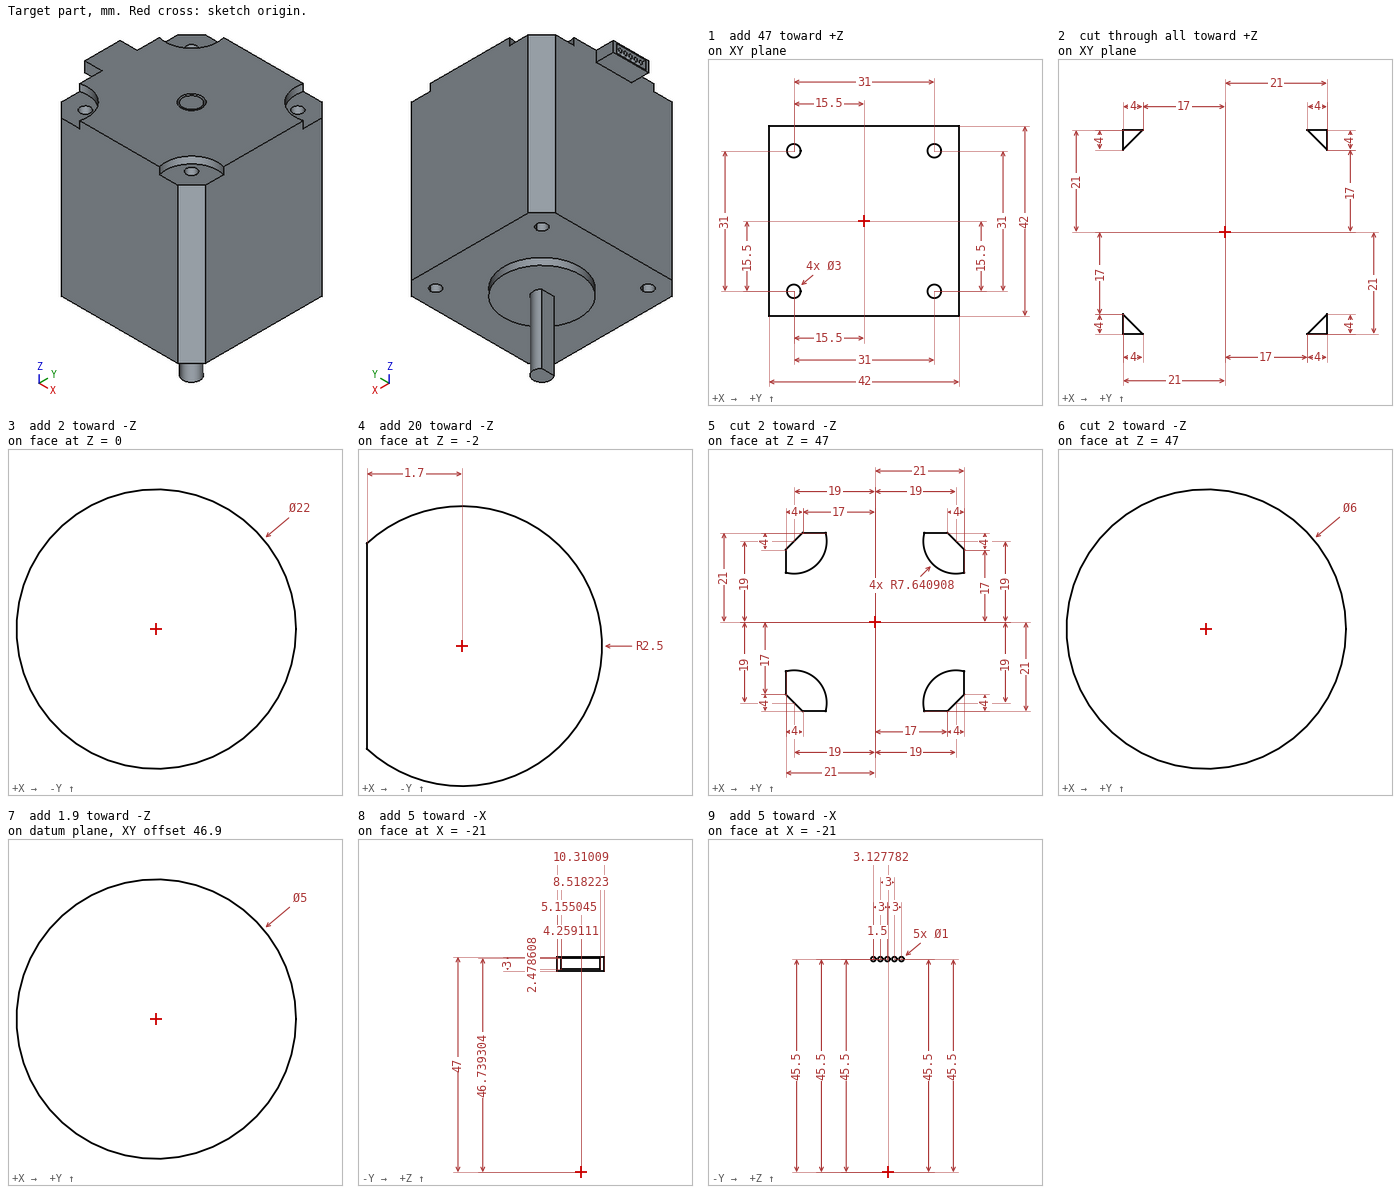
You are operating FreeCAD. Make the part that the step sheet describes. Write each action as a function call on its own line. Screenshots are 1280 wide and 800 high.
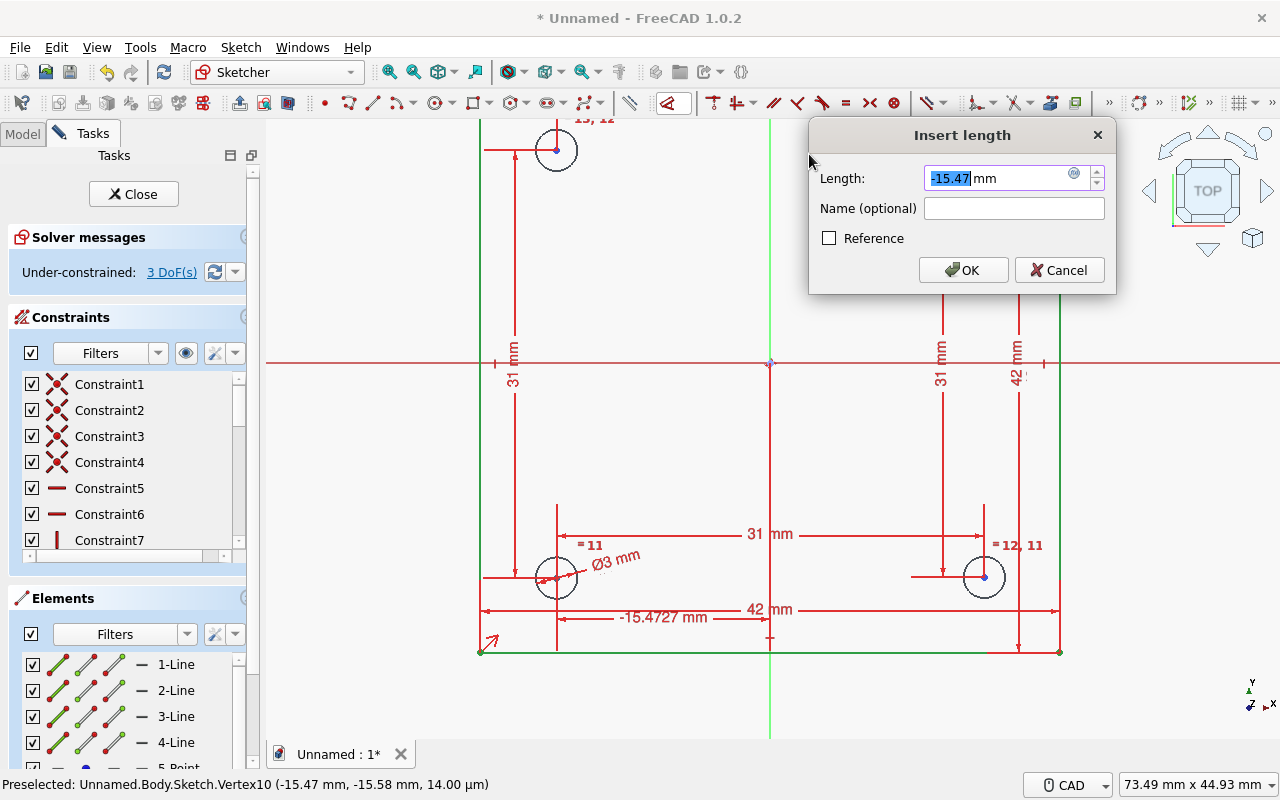
text(-15.5)
key(Return)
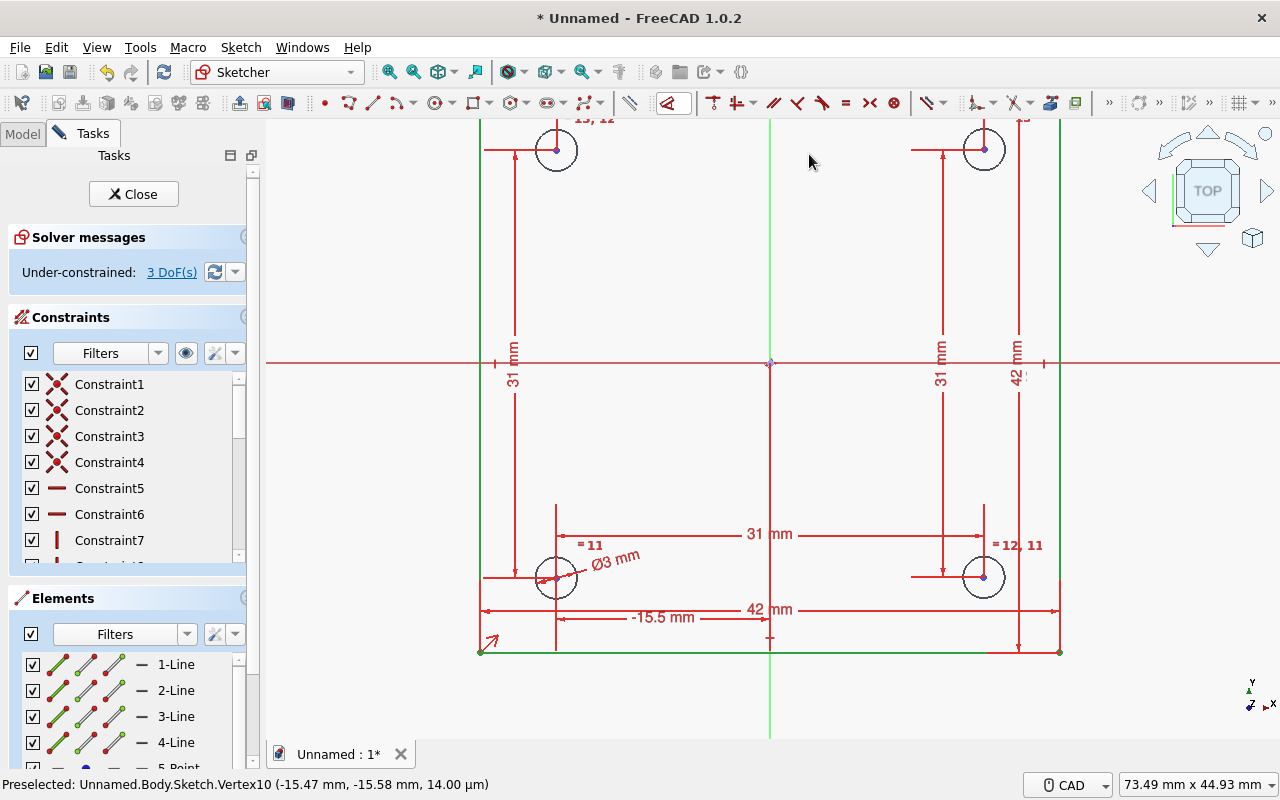
click(556, 578)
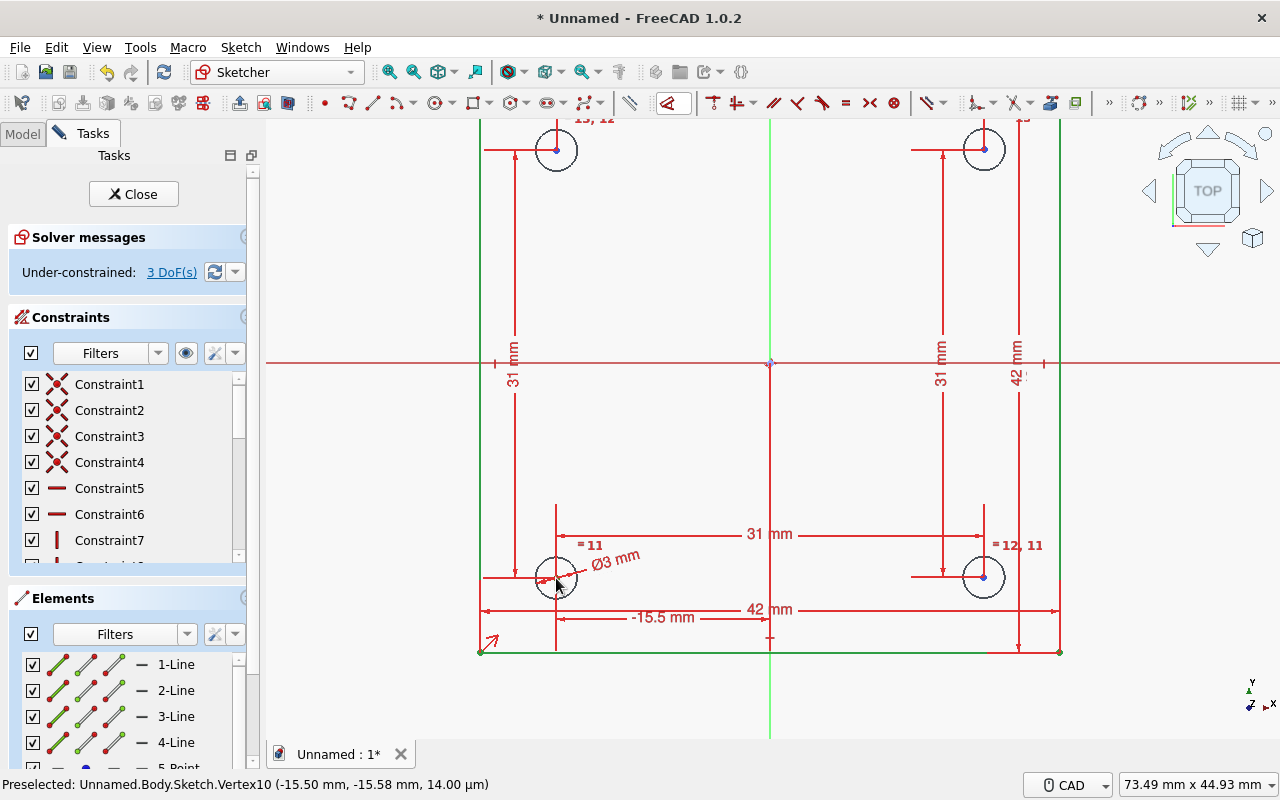
key(i)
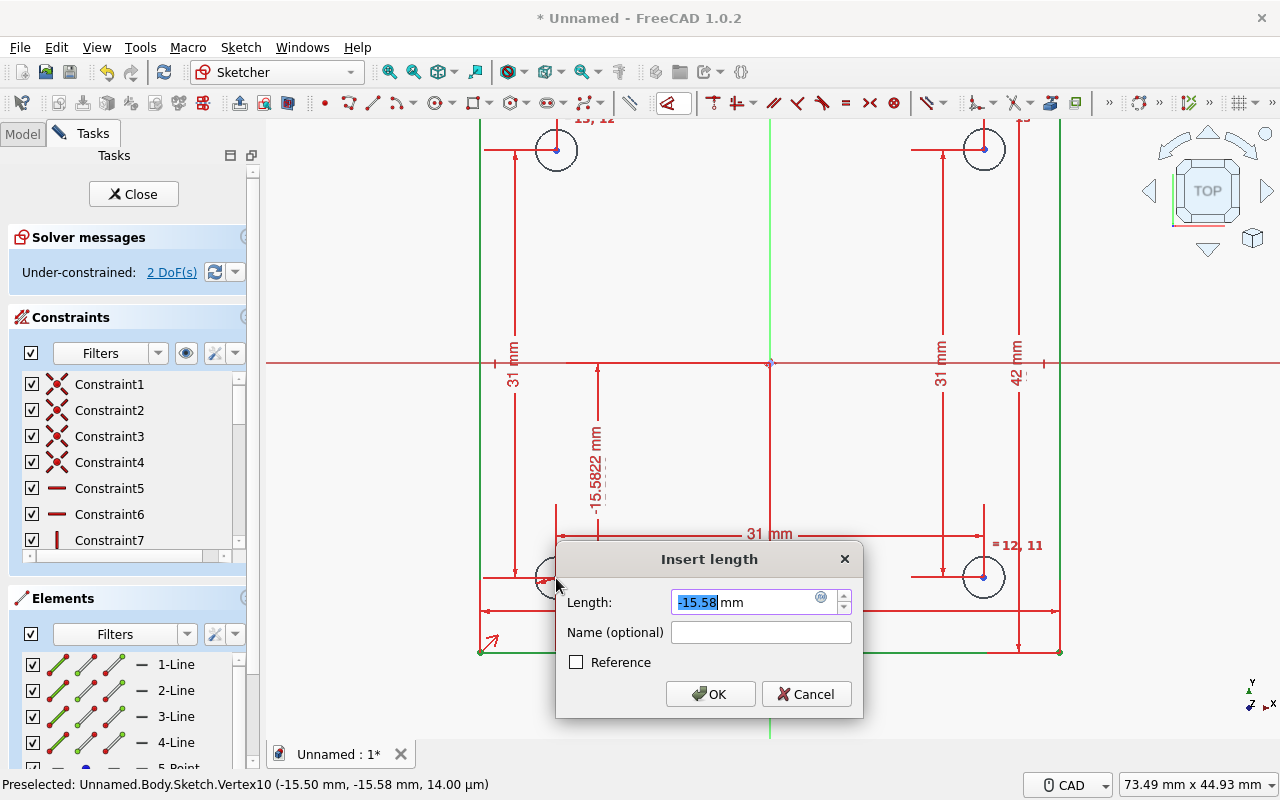
text(-15.5)
key(Return)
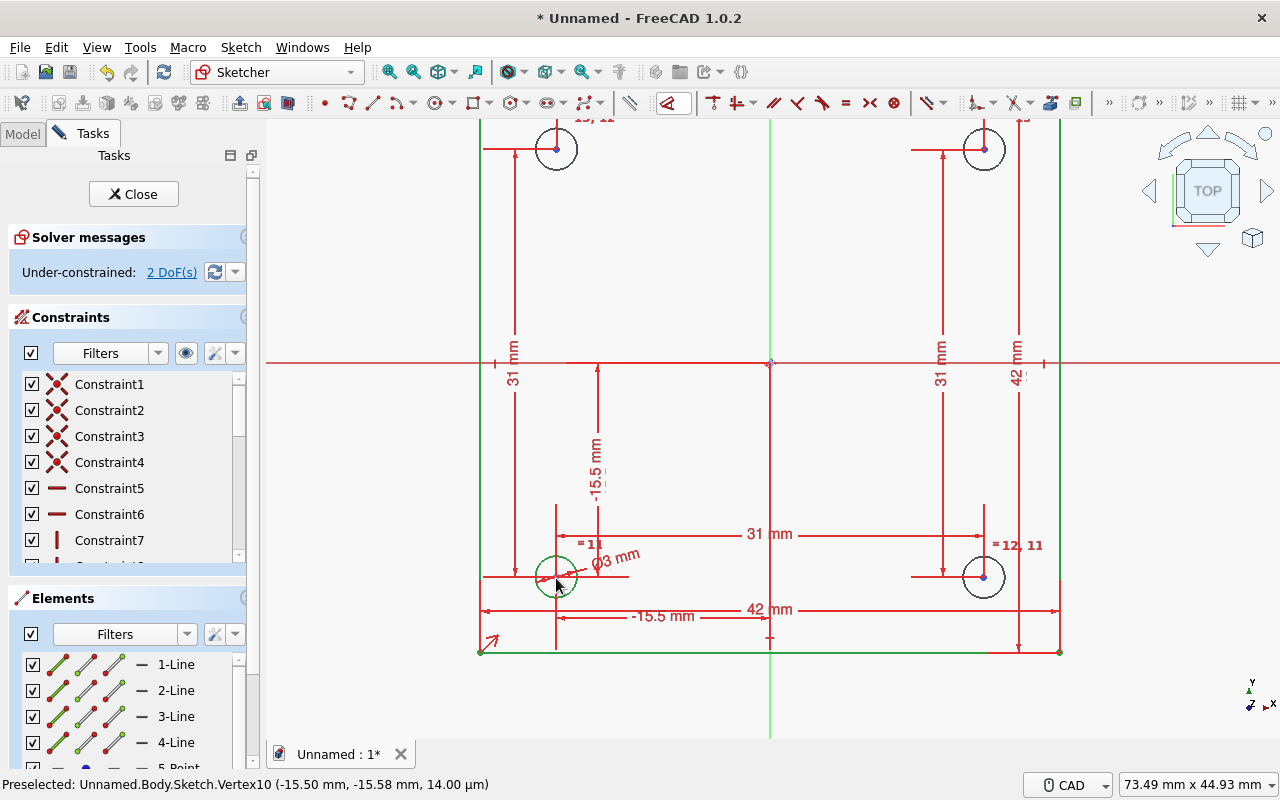
click(984, 577)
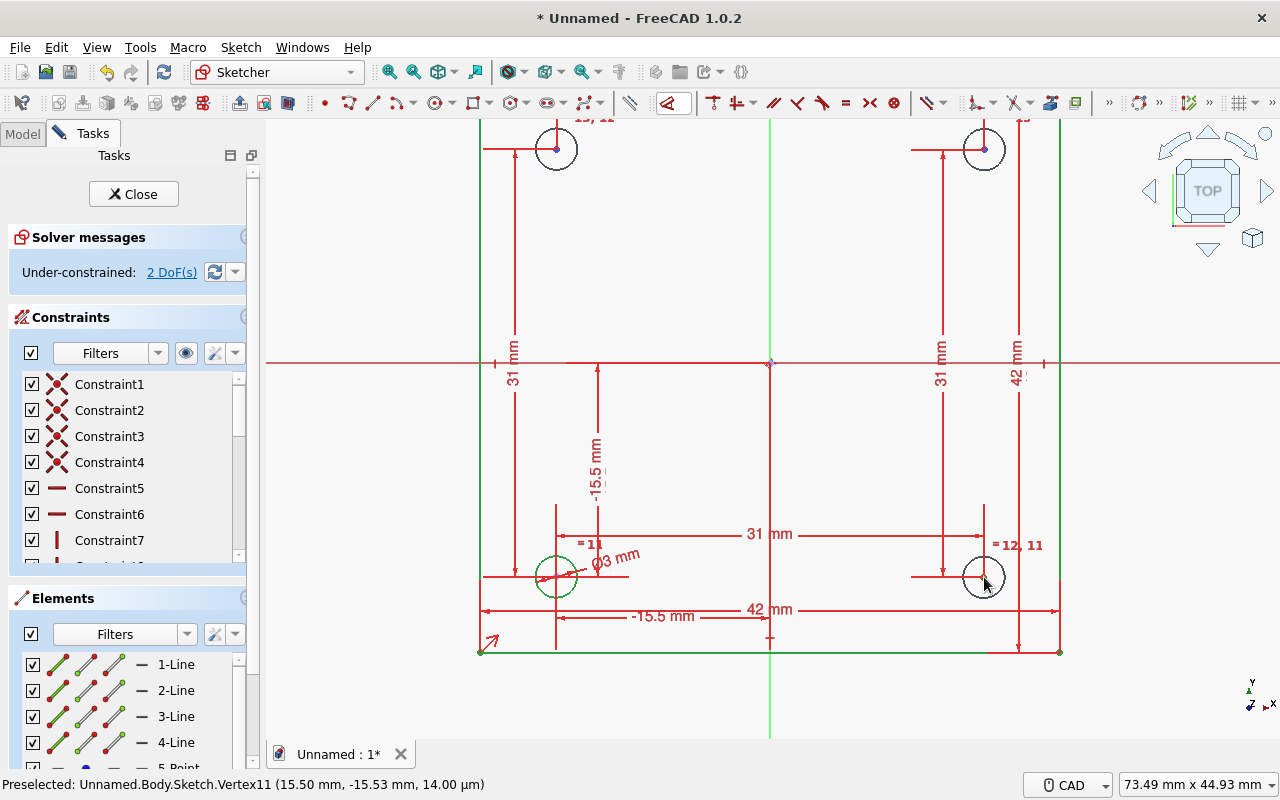
click(686, 104)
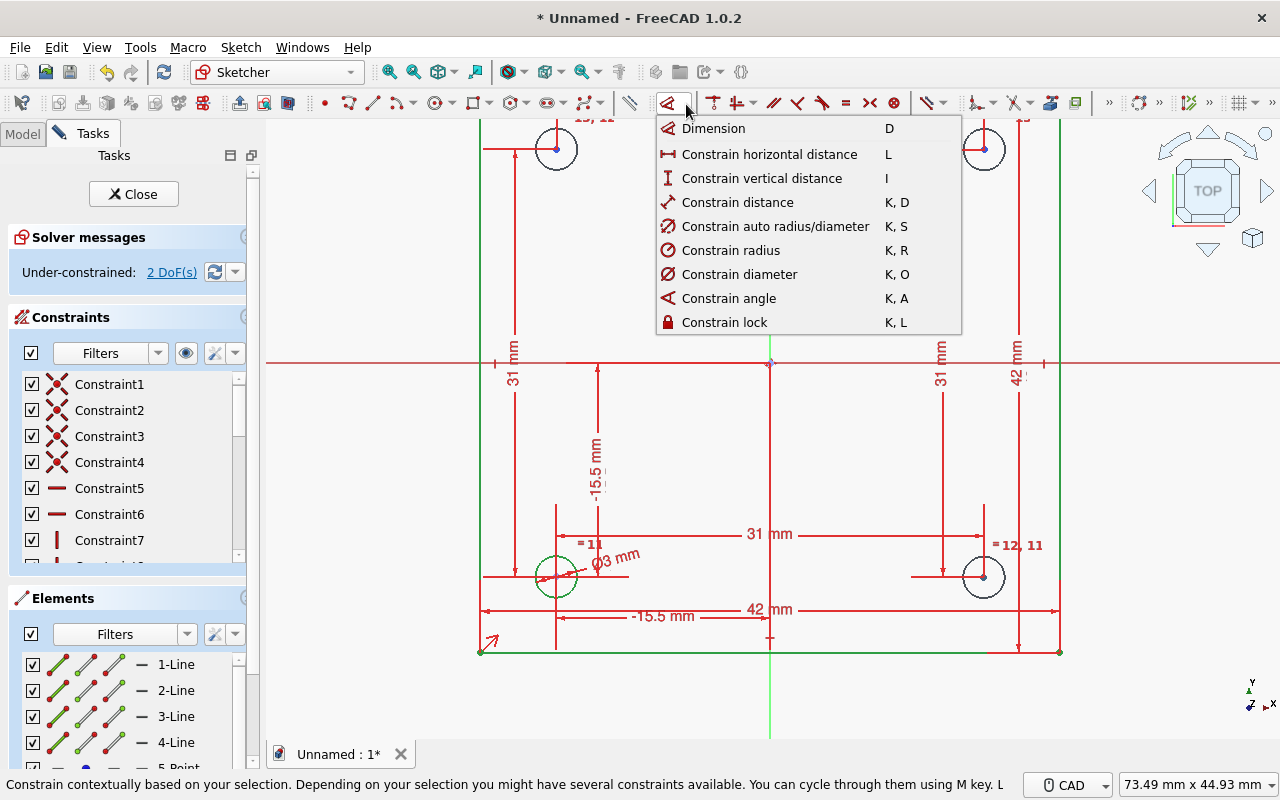
click(809, 178)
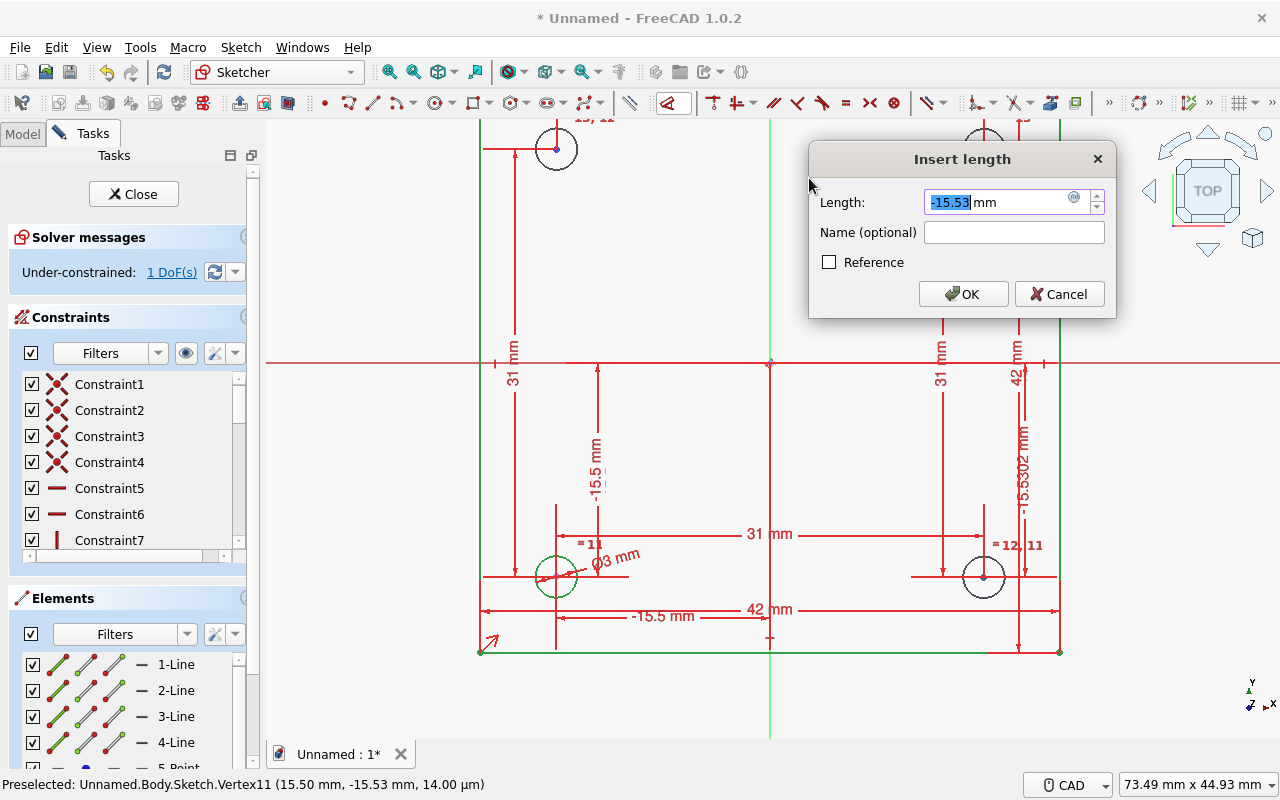
text(-15.5)
key(Return)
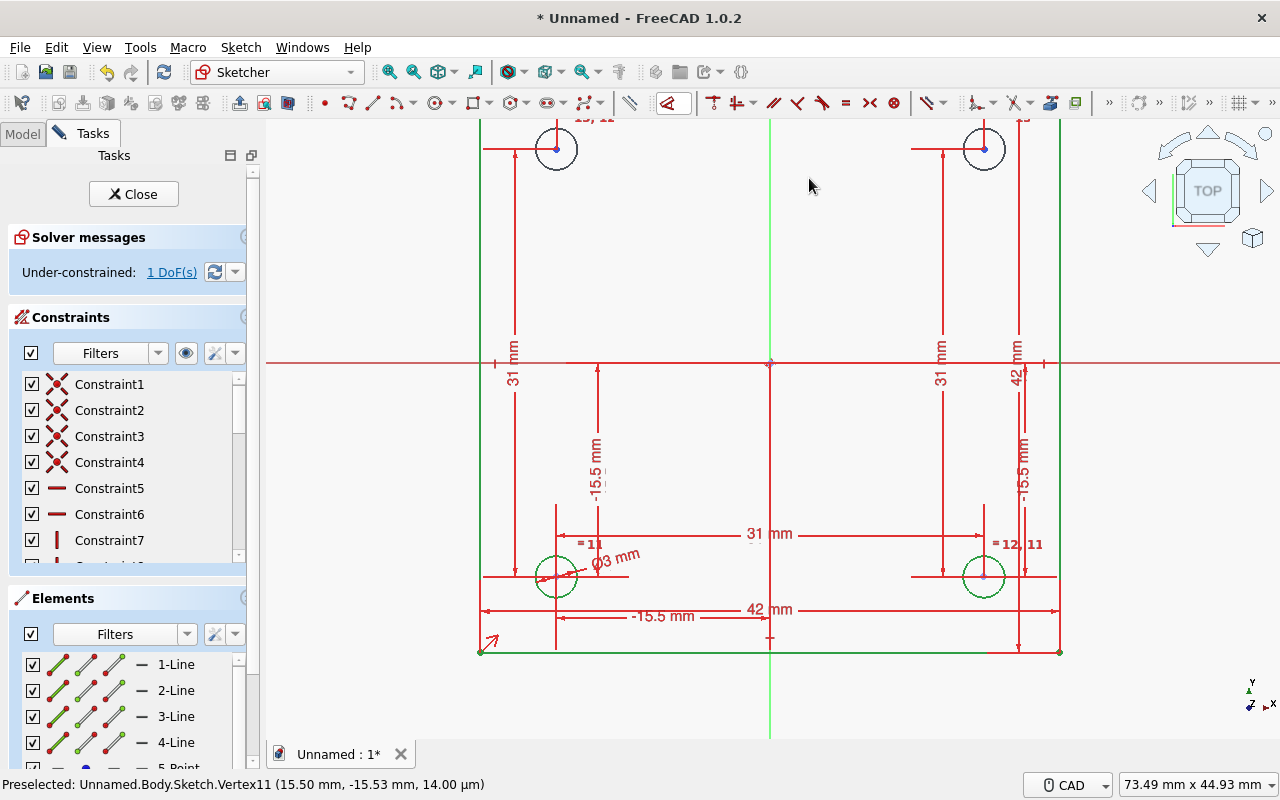
click(557, 149)